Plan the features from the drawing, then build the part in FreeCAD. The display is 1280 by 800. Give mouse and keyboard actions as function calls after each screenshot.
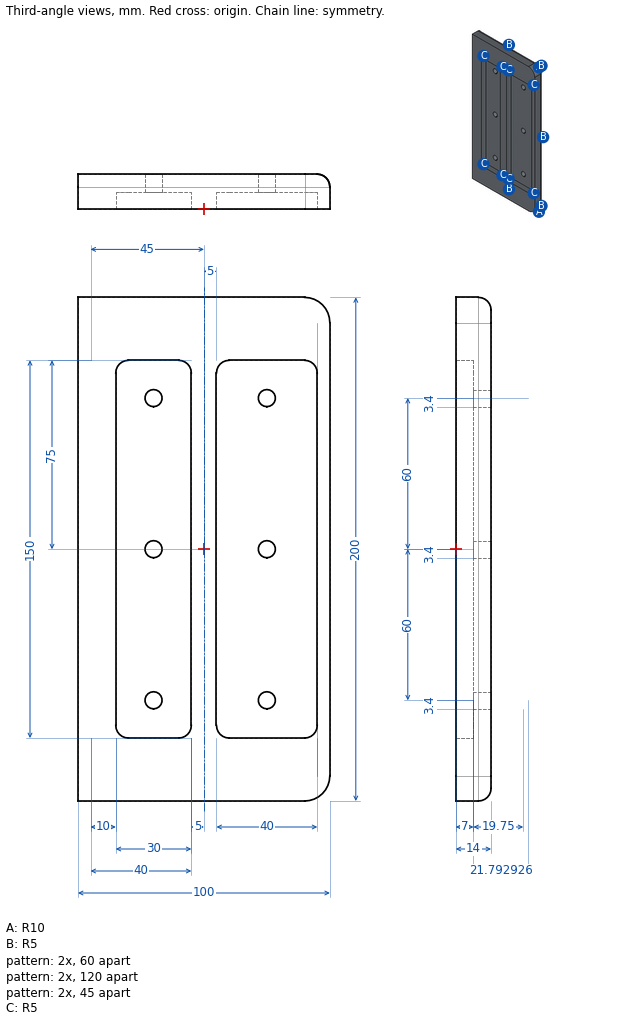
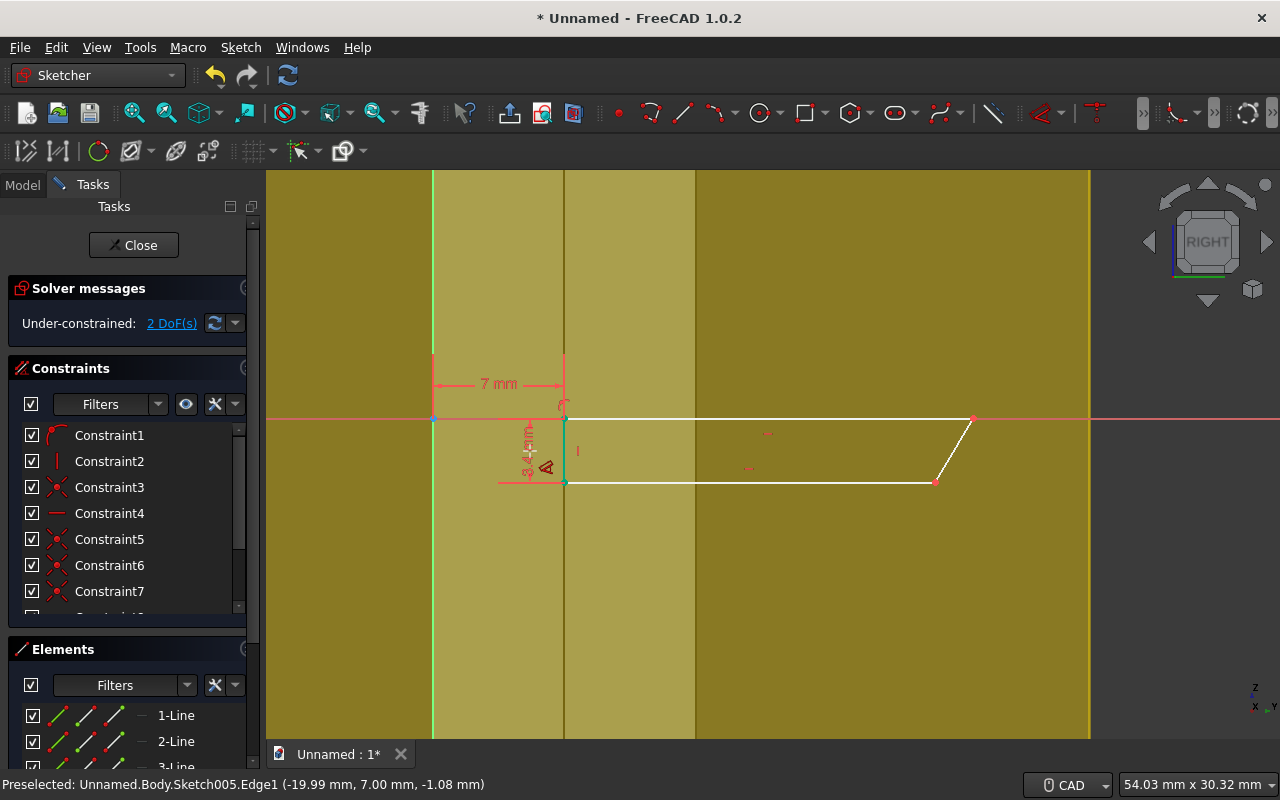
click(676, 483)
click(750, 517)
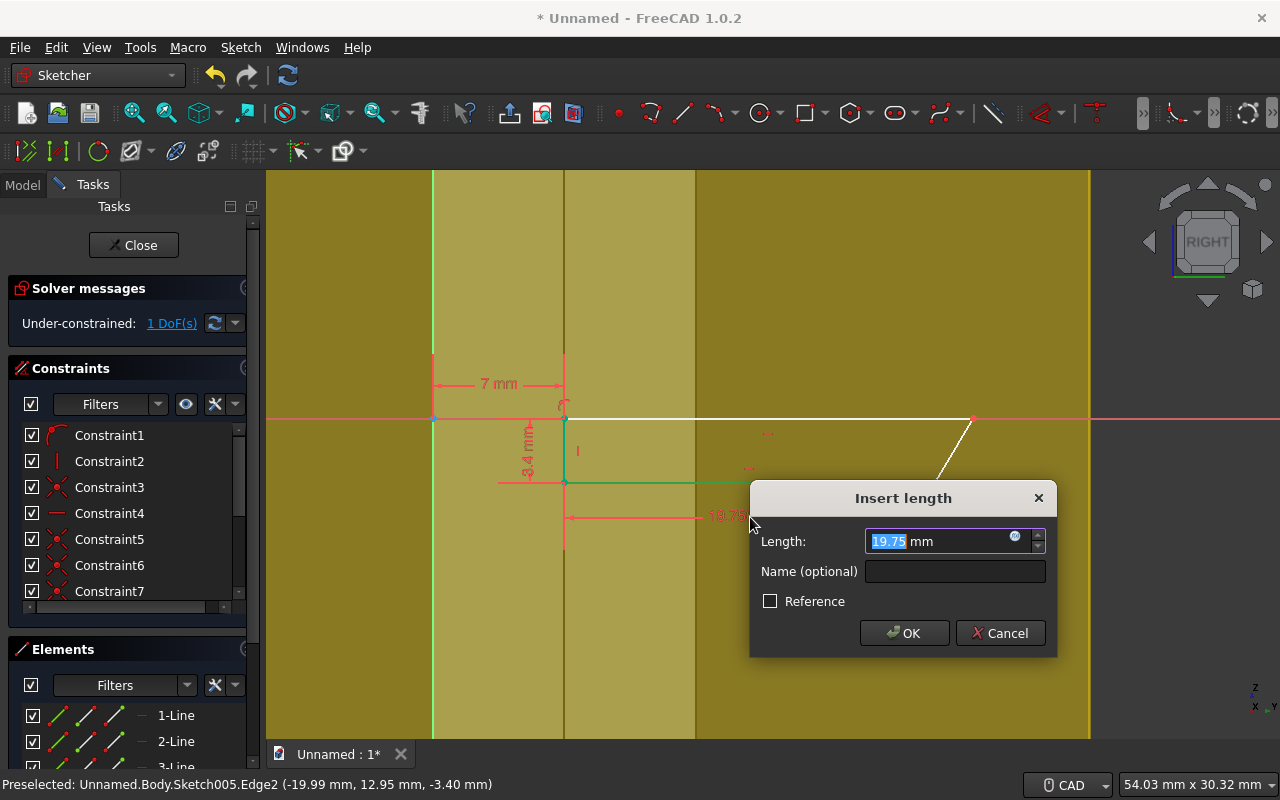
text(19.75)
key(Return)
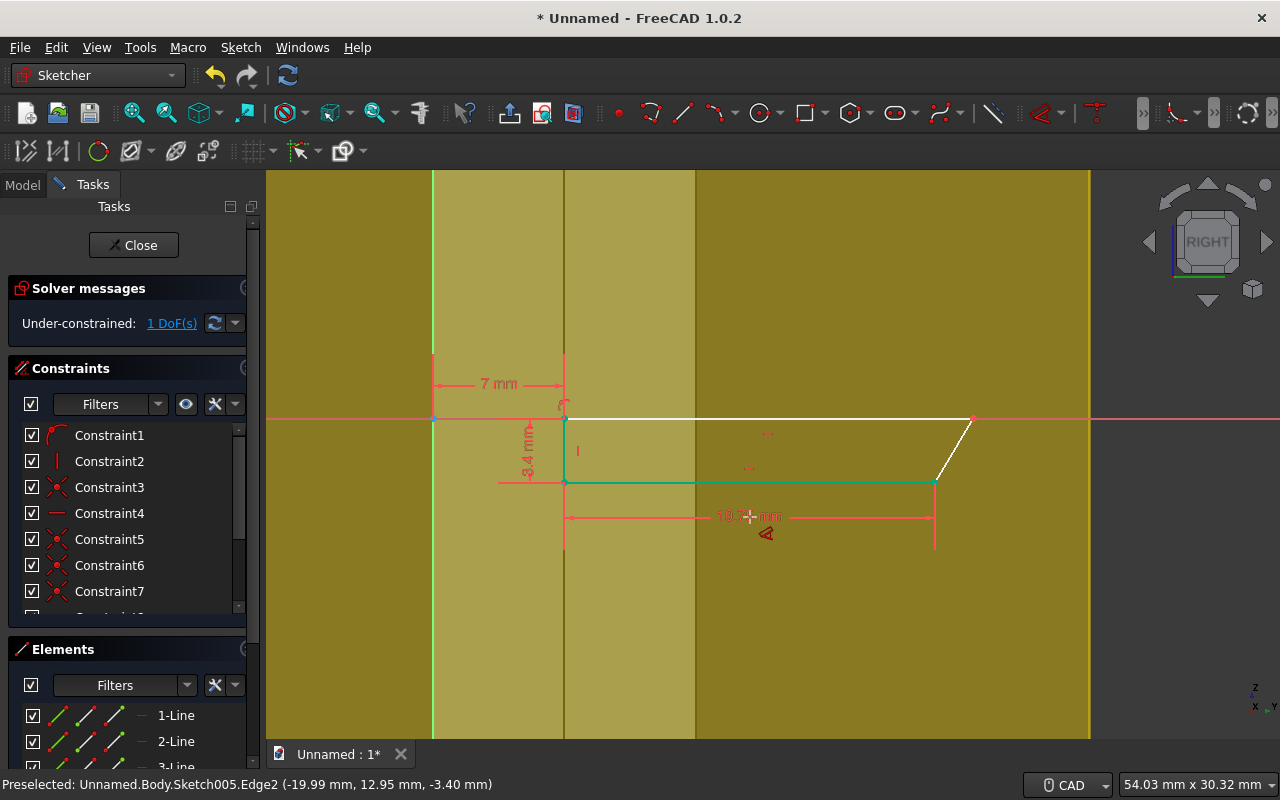
click(850, 419)
click(769, 385)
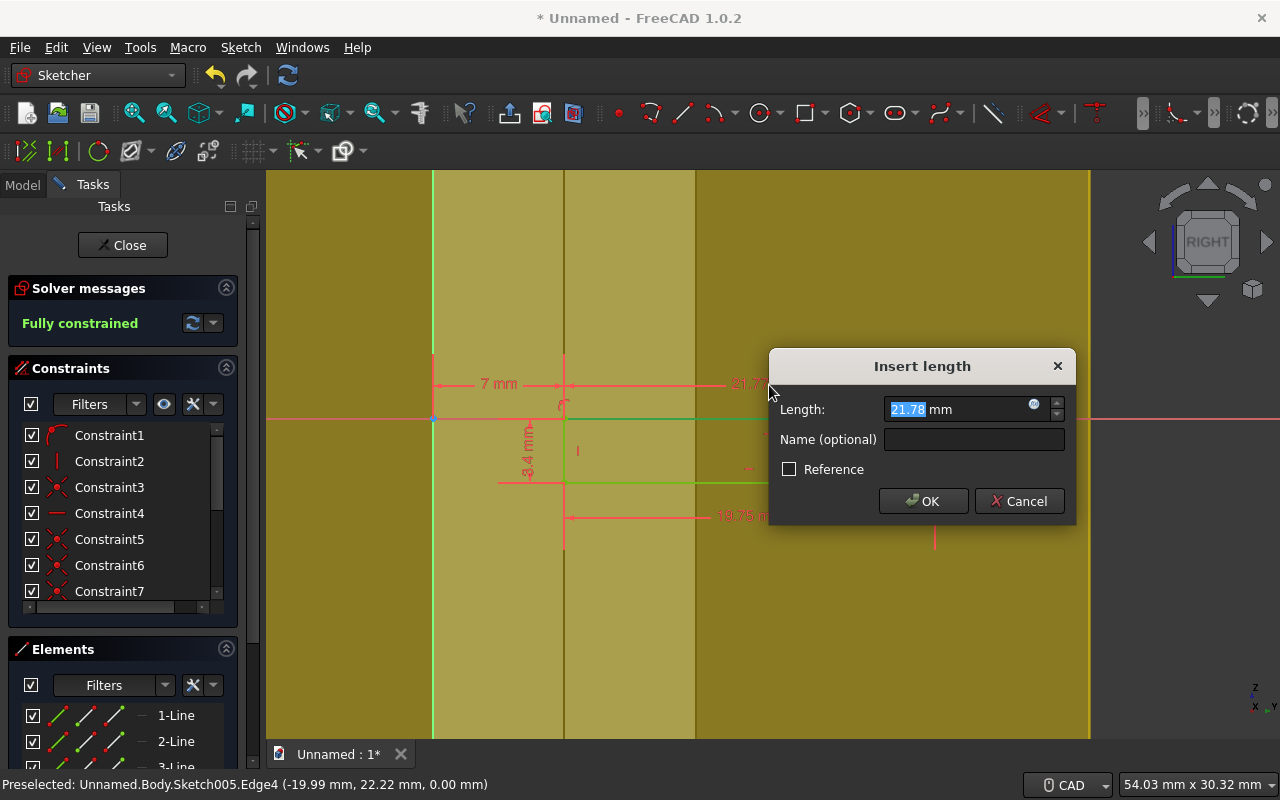
text(21.792926)
key(Return)
key(Escape)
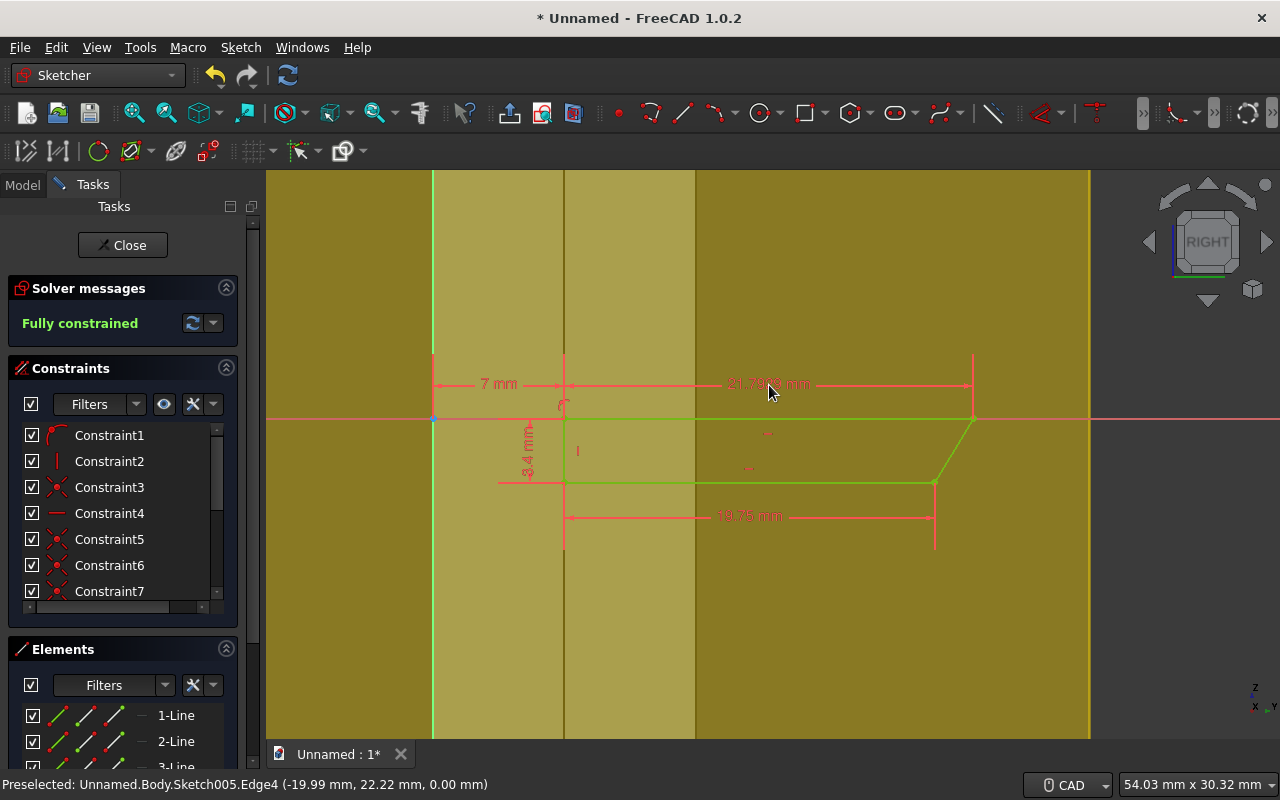
click(123, 245)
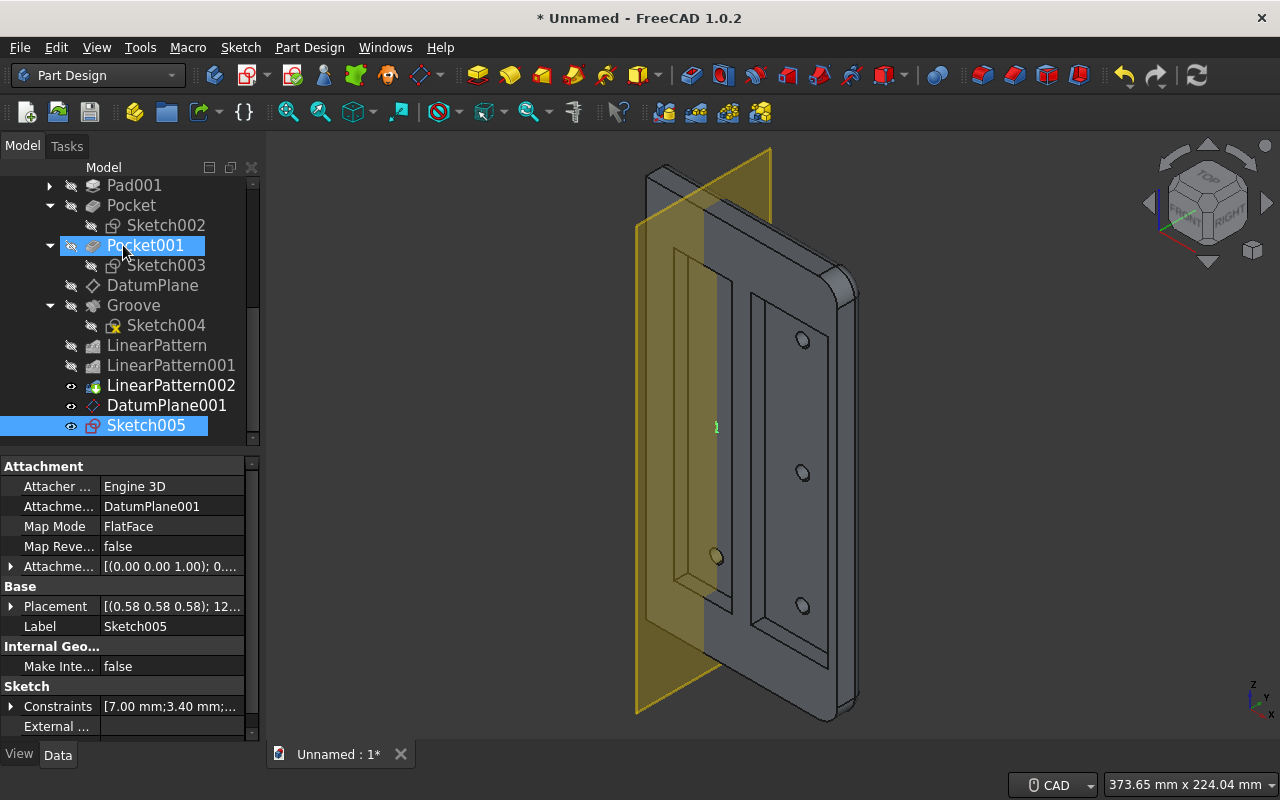
click(756, 76)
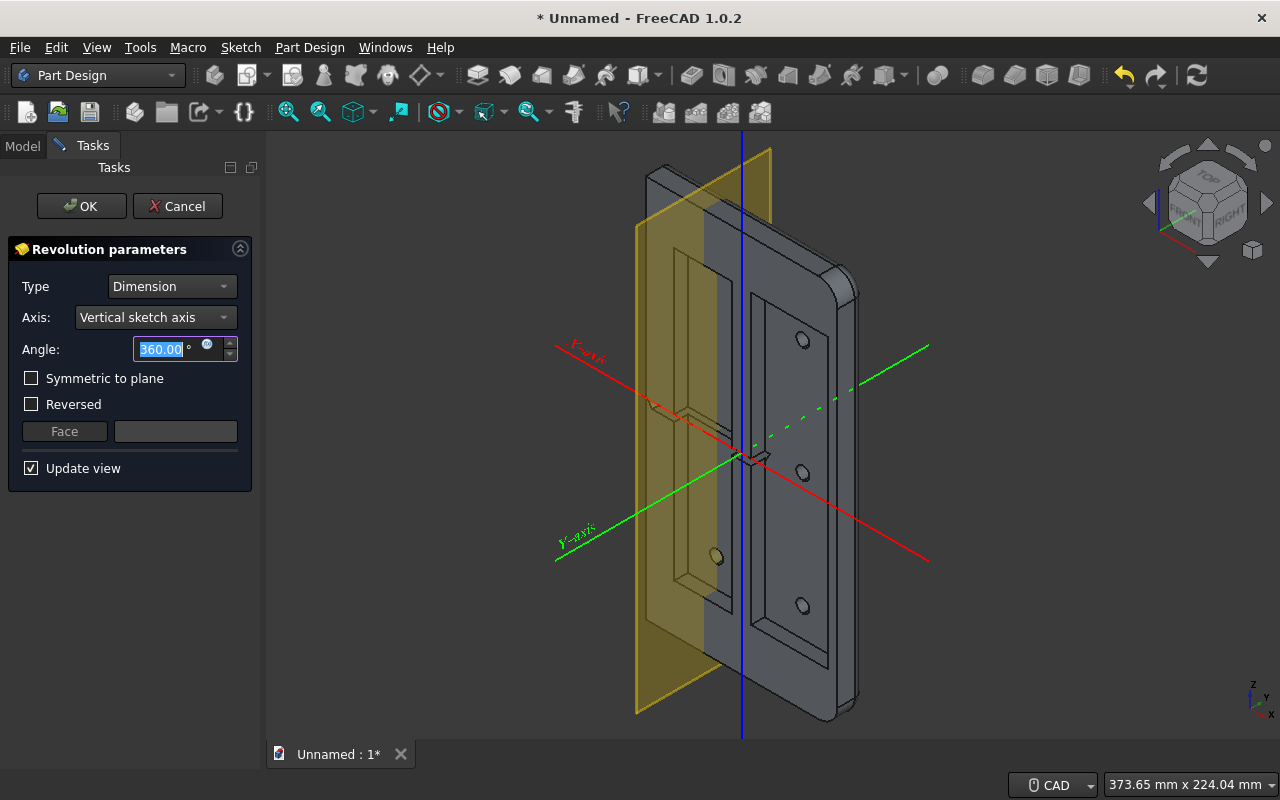
click(156, 318)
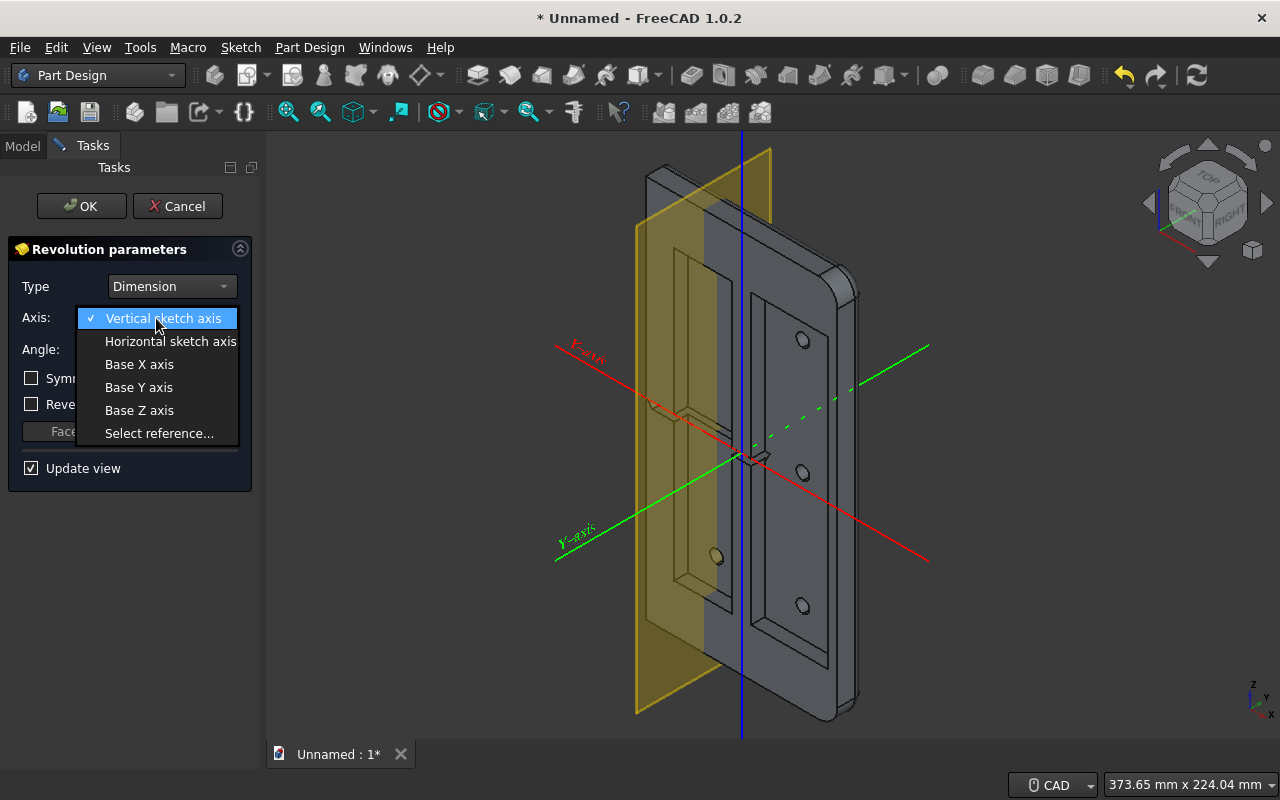
click(156, 342)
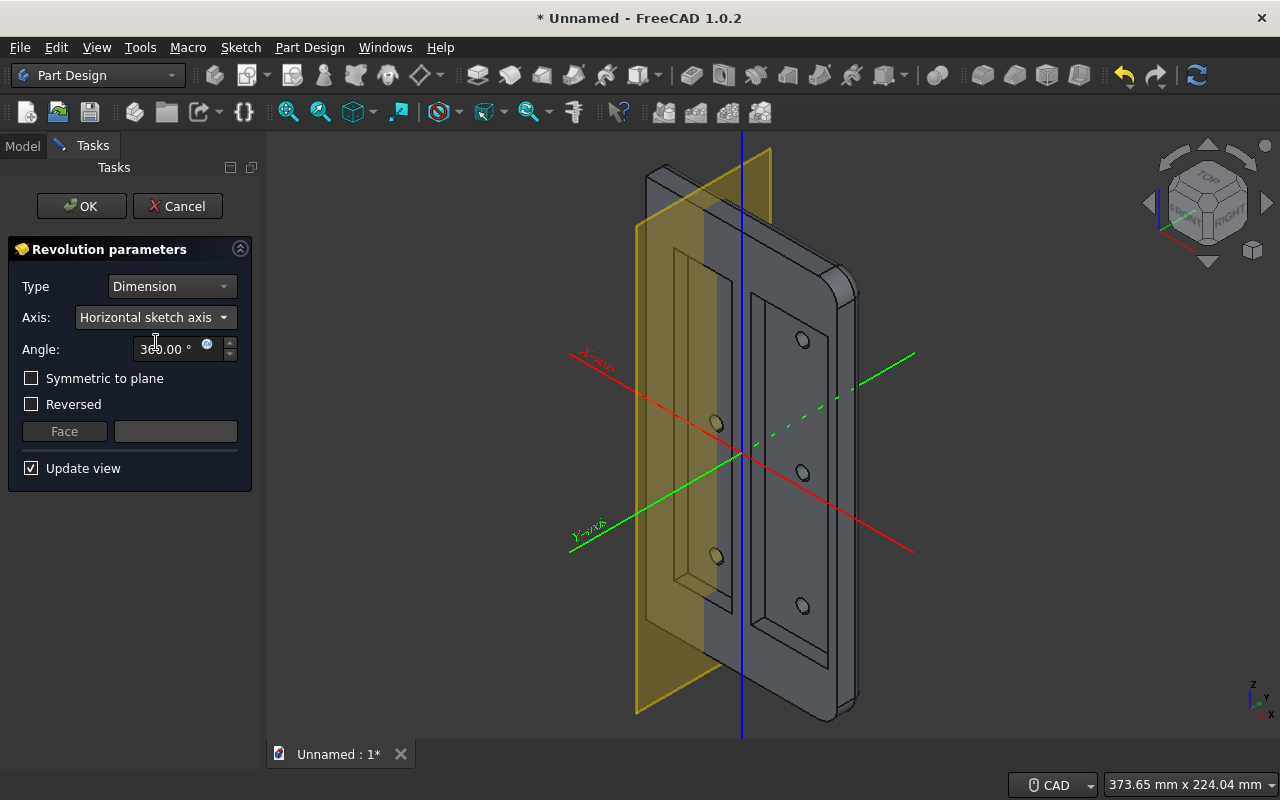
click(82, 206)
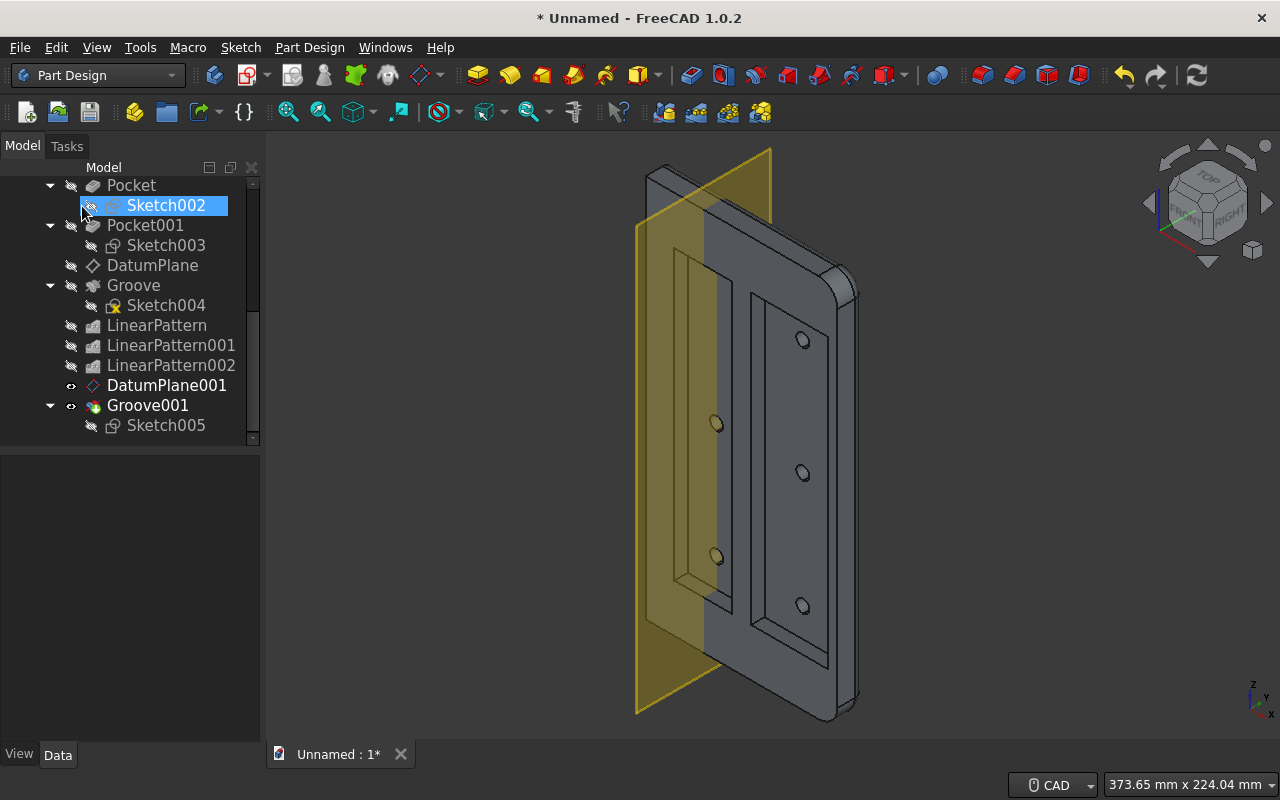
click(116, 386)
key(space)